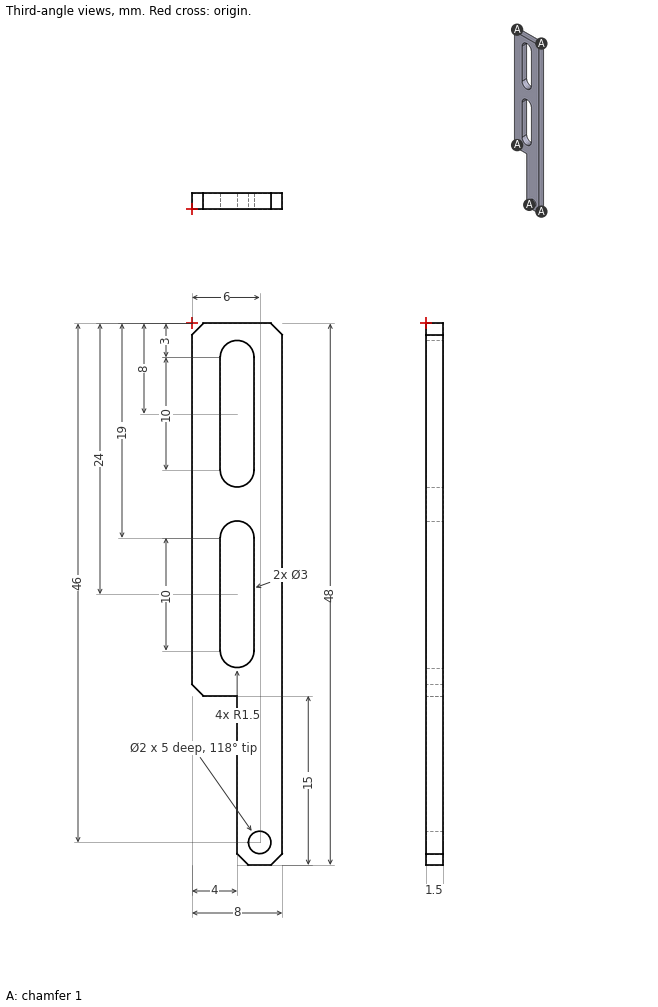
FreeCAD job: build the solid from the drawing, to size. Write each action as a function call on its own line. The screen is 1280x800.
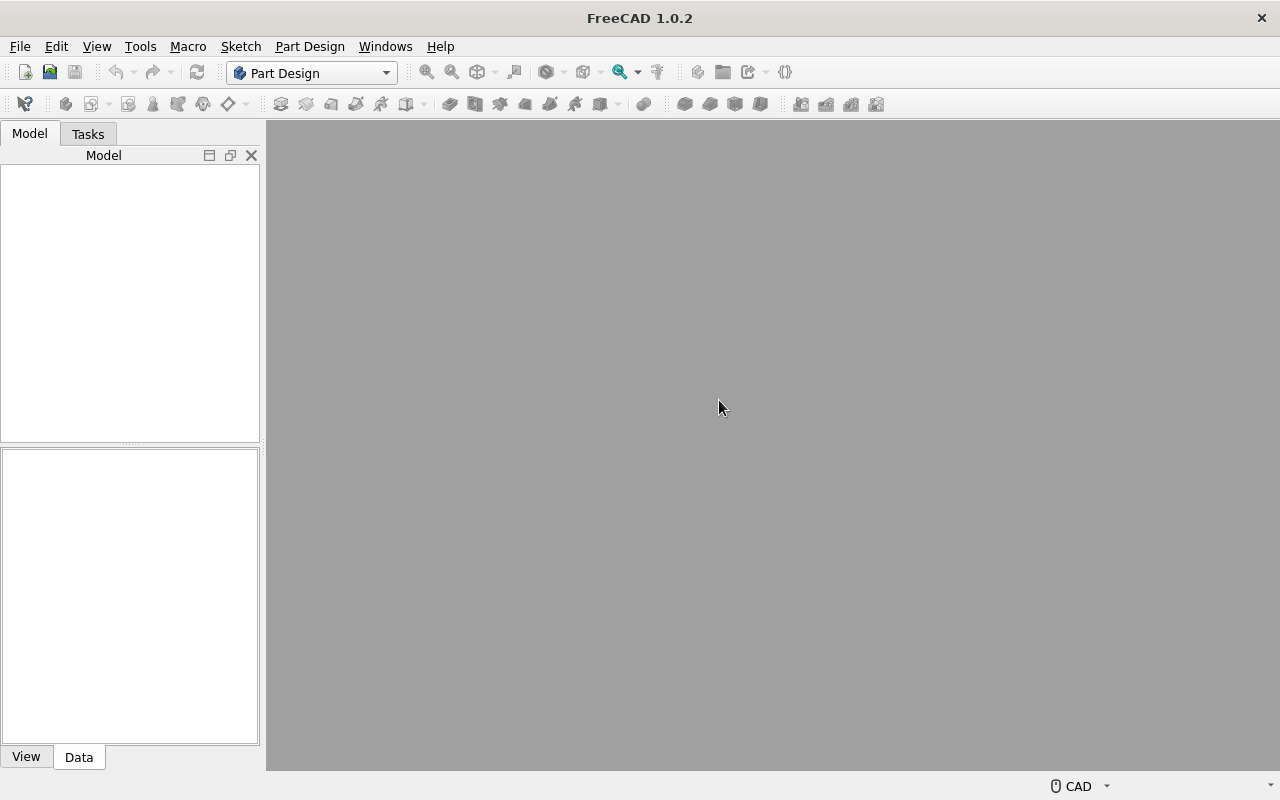
click(25, 72)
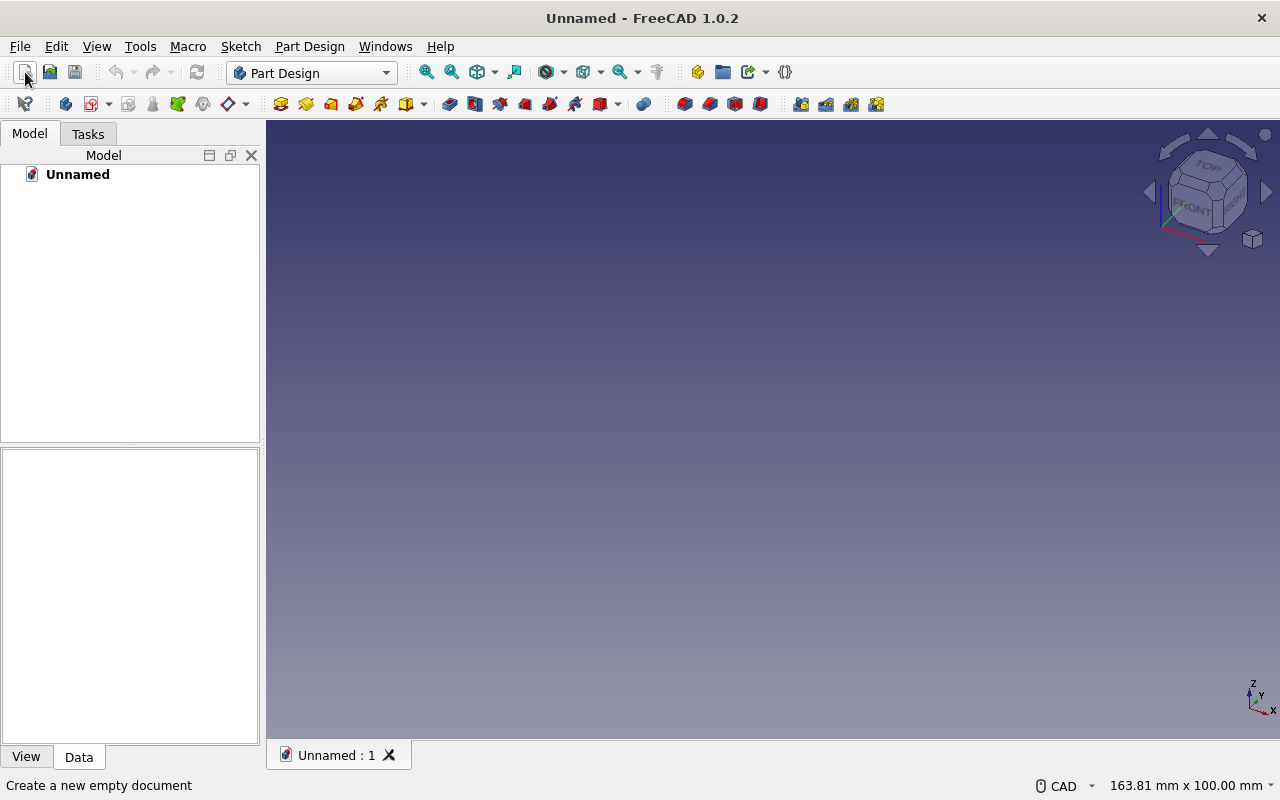
click(90, 104)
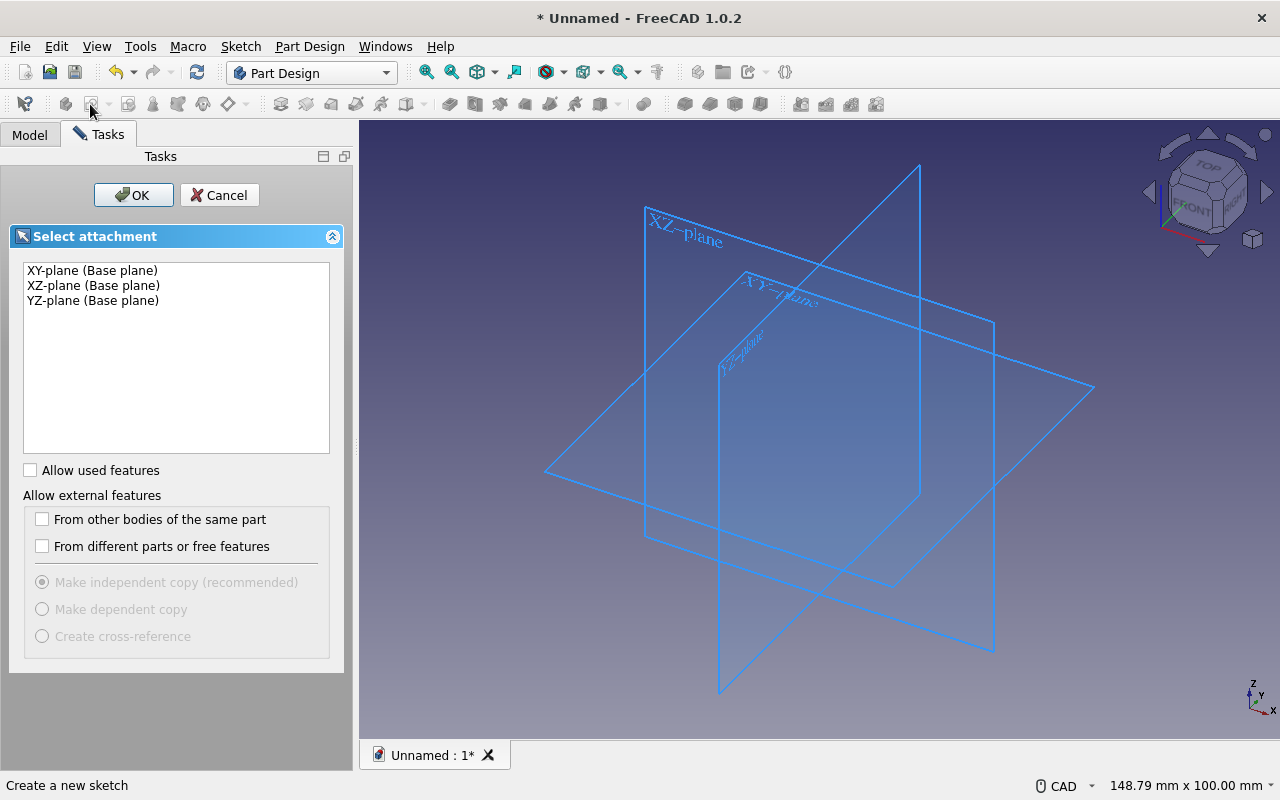
click(84, 286)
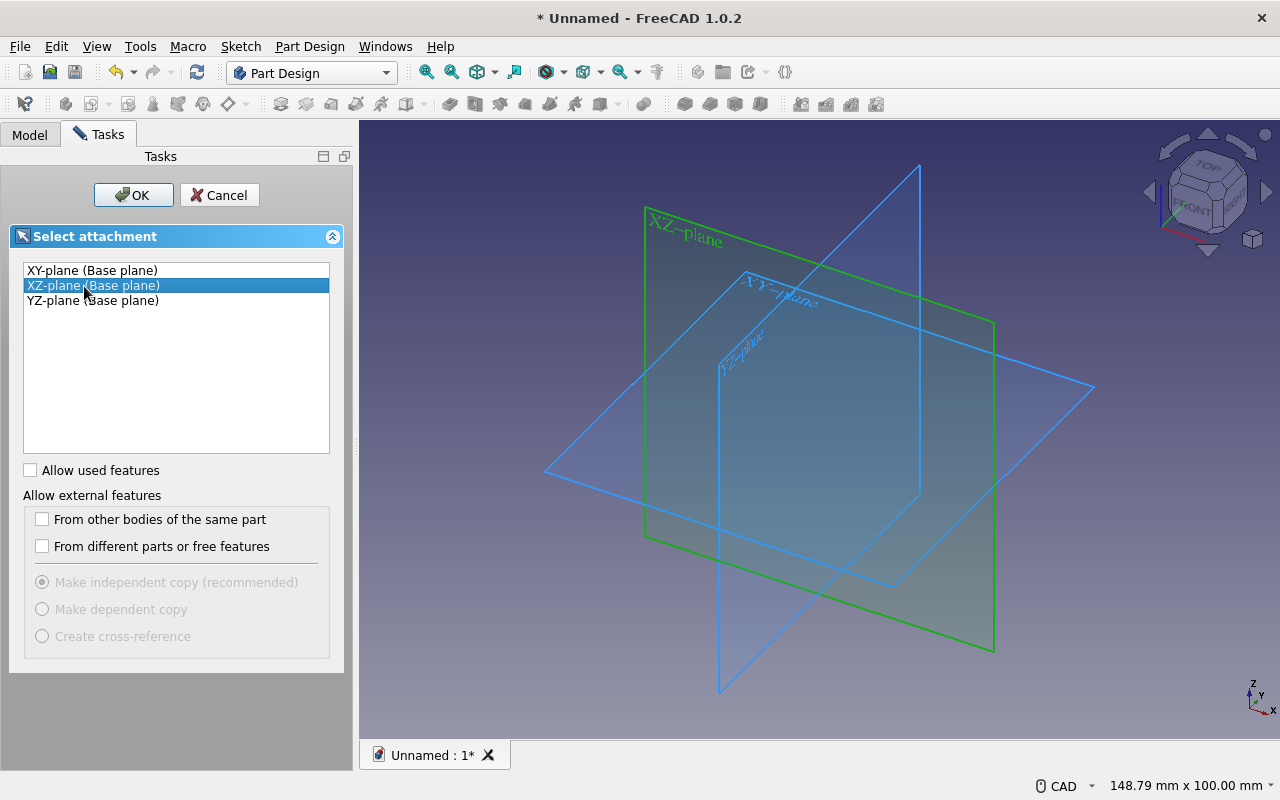
click(134, 195)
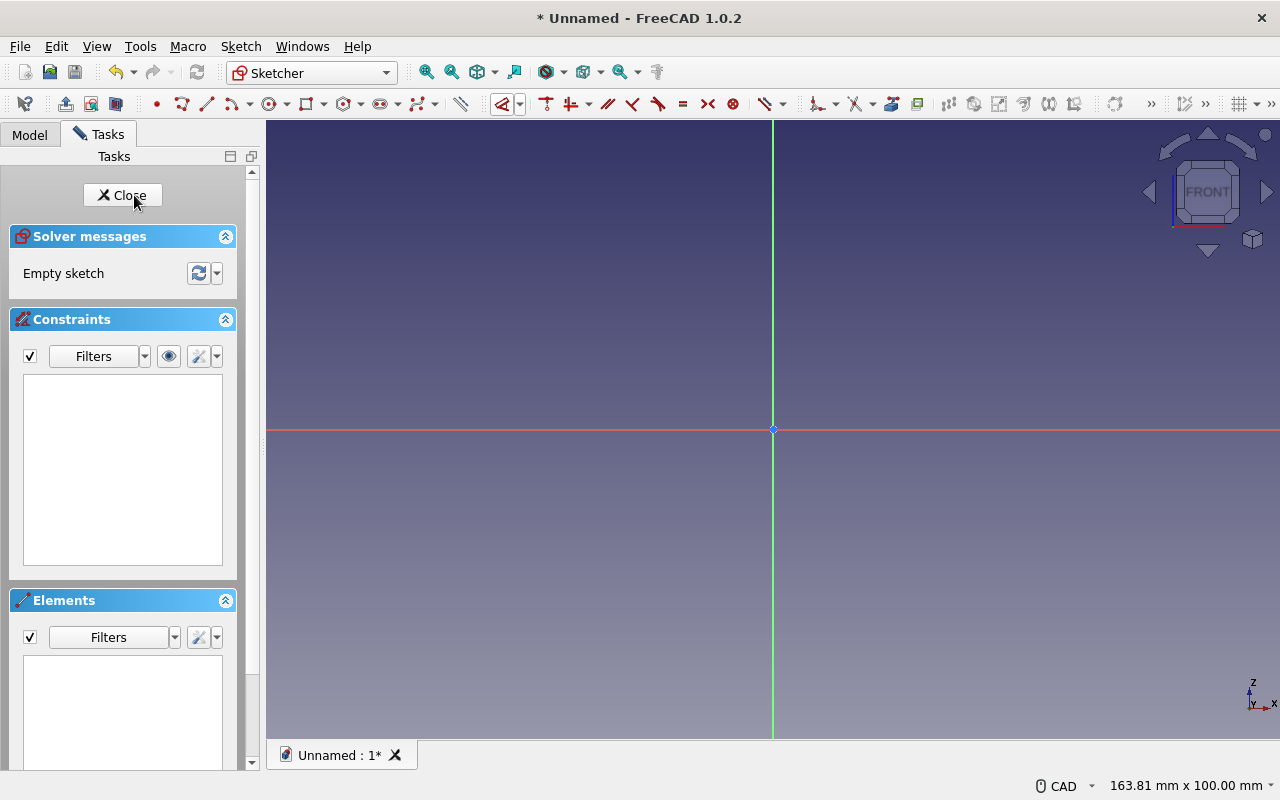
scroll(294, 148, down, 1)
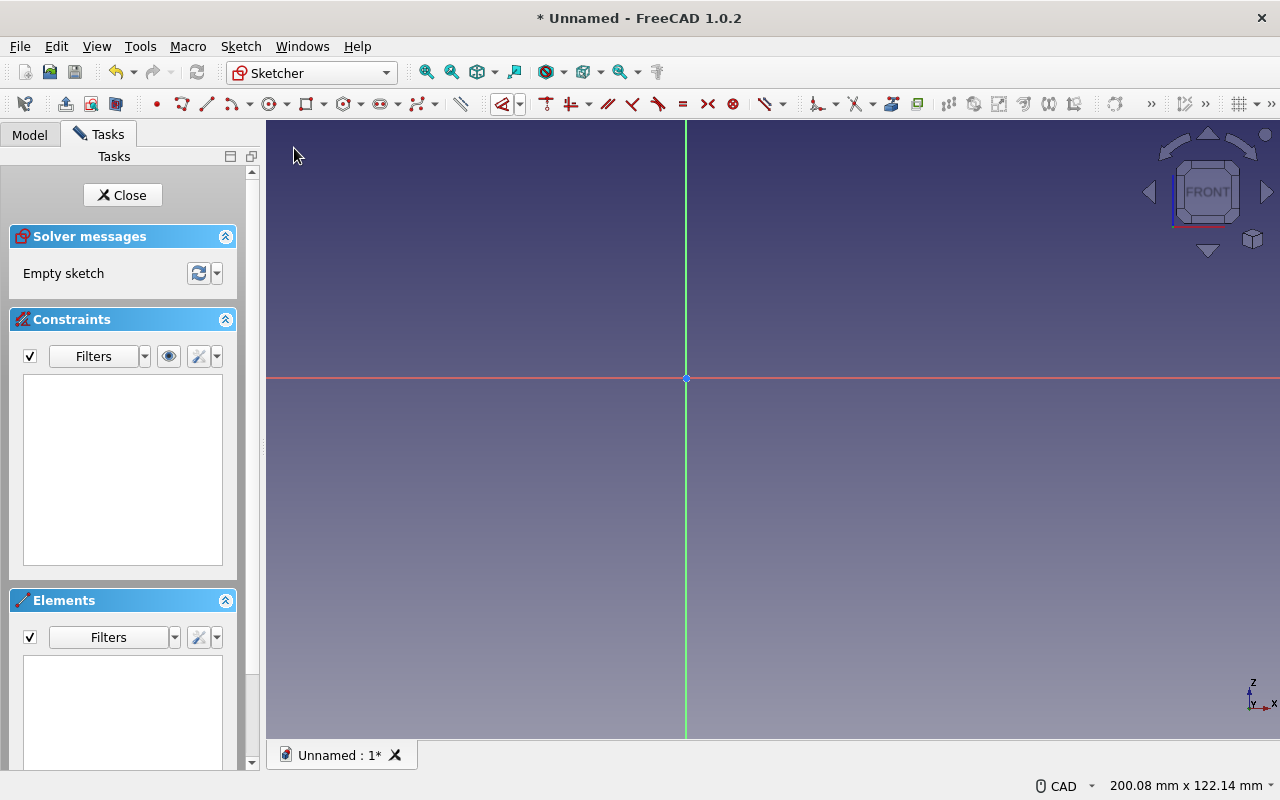
scroll(710, 644, up, 2)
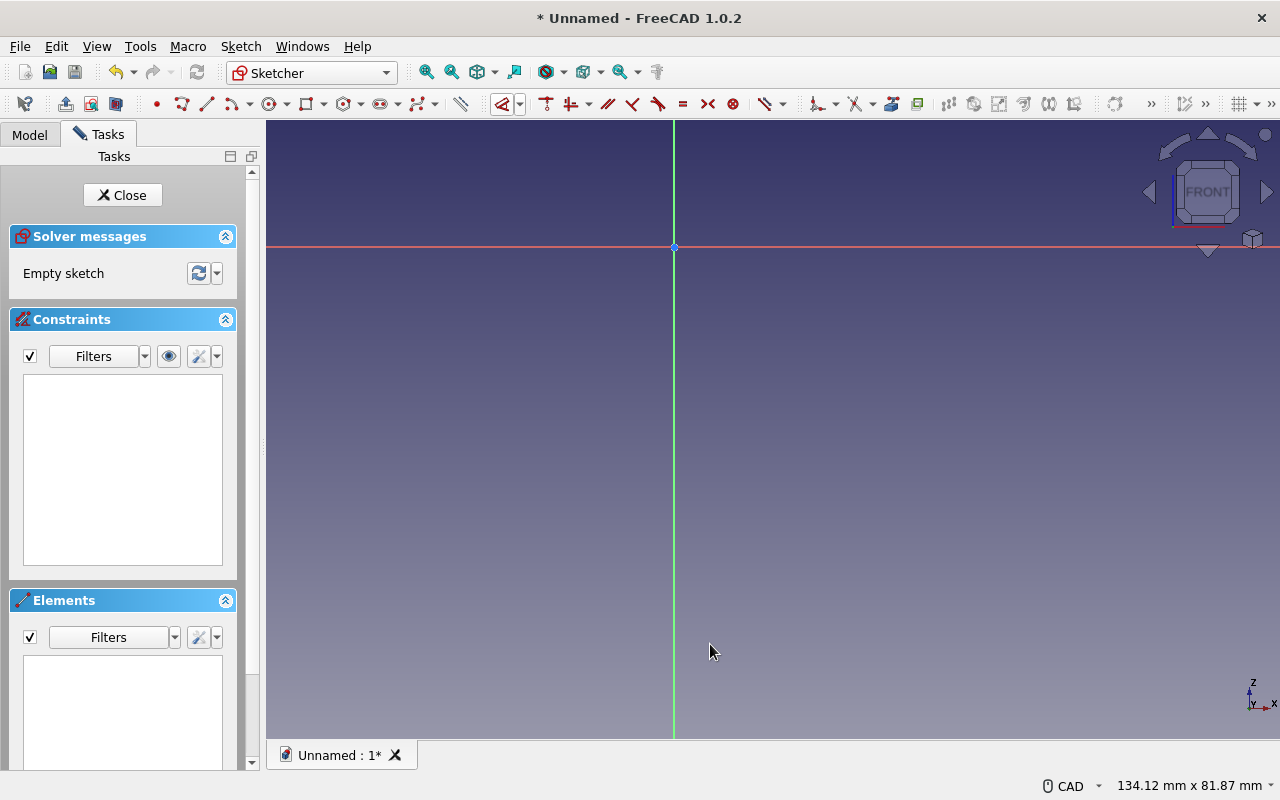
key(g)
key(r)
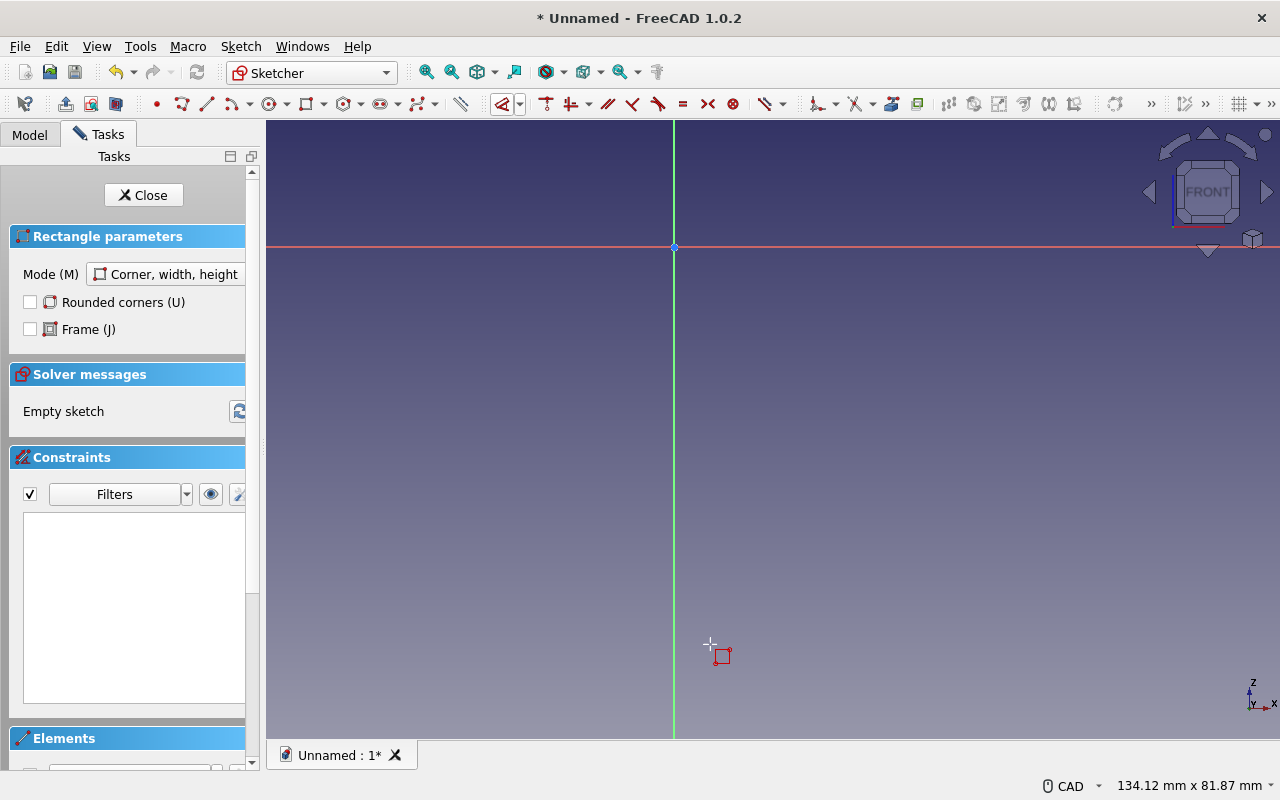
click(674, 247)
move(735, 610)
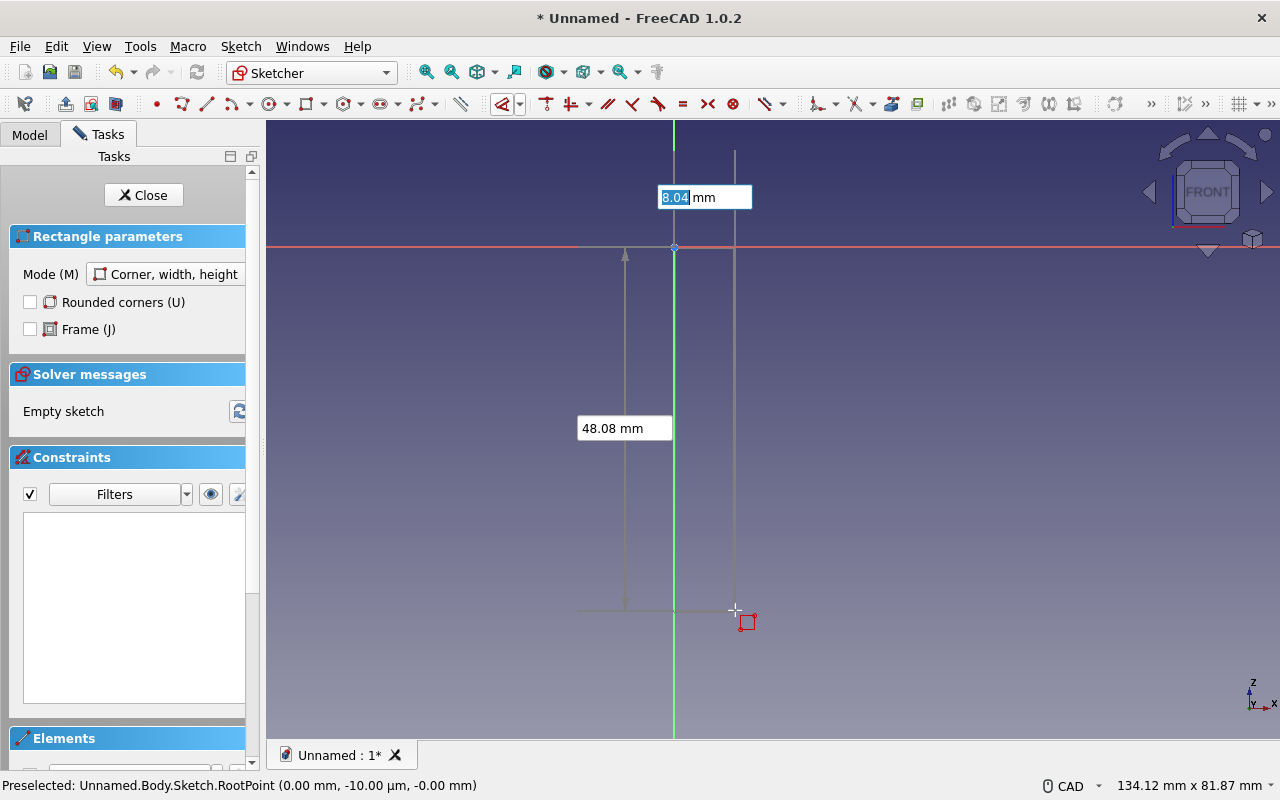
text(8)
key(Tab)
text(48)
key(Return)
key(Escape)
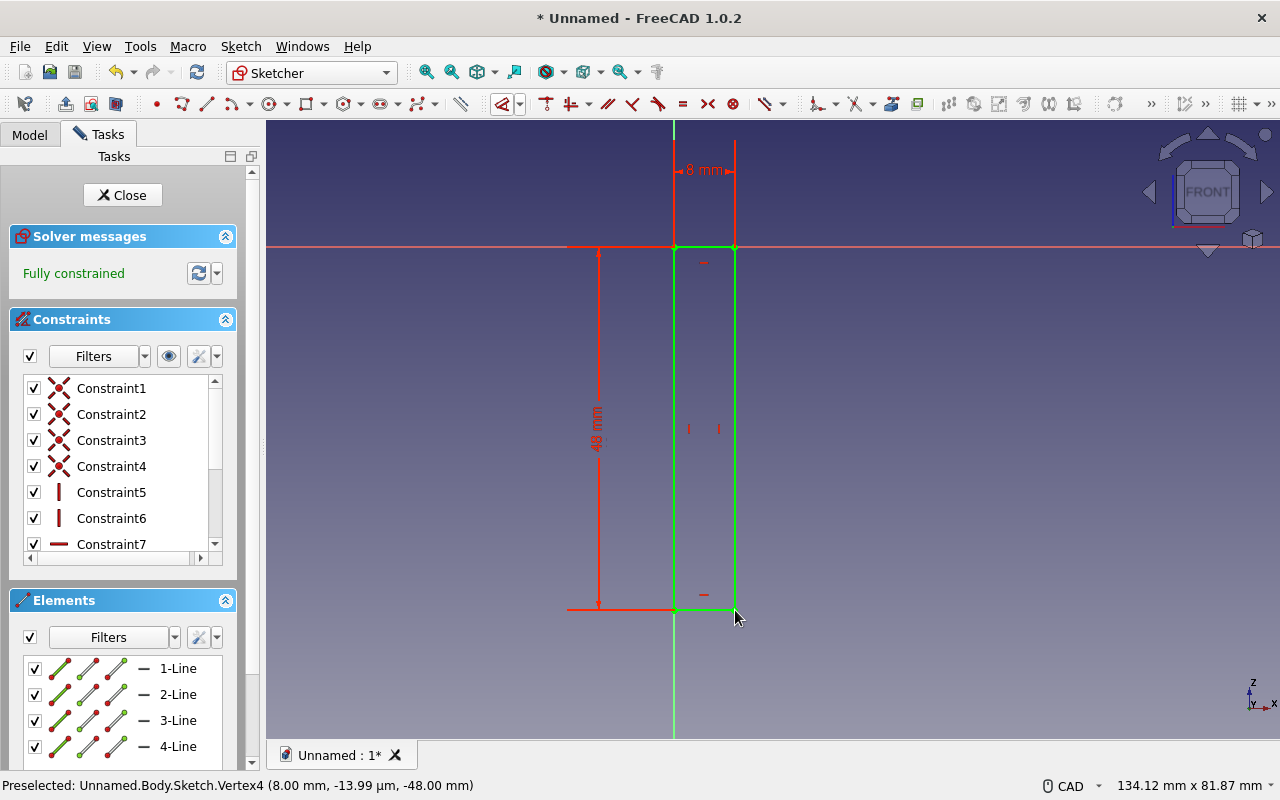
click(123, 195)